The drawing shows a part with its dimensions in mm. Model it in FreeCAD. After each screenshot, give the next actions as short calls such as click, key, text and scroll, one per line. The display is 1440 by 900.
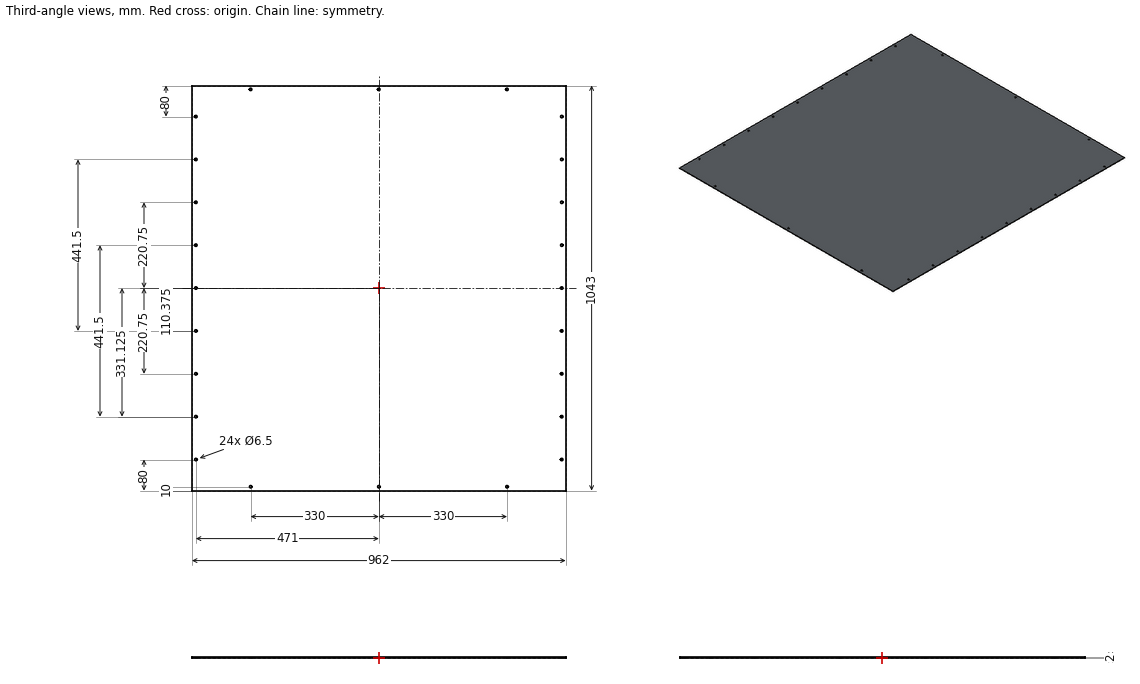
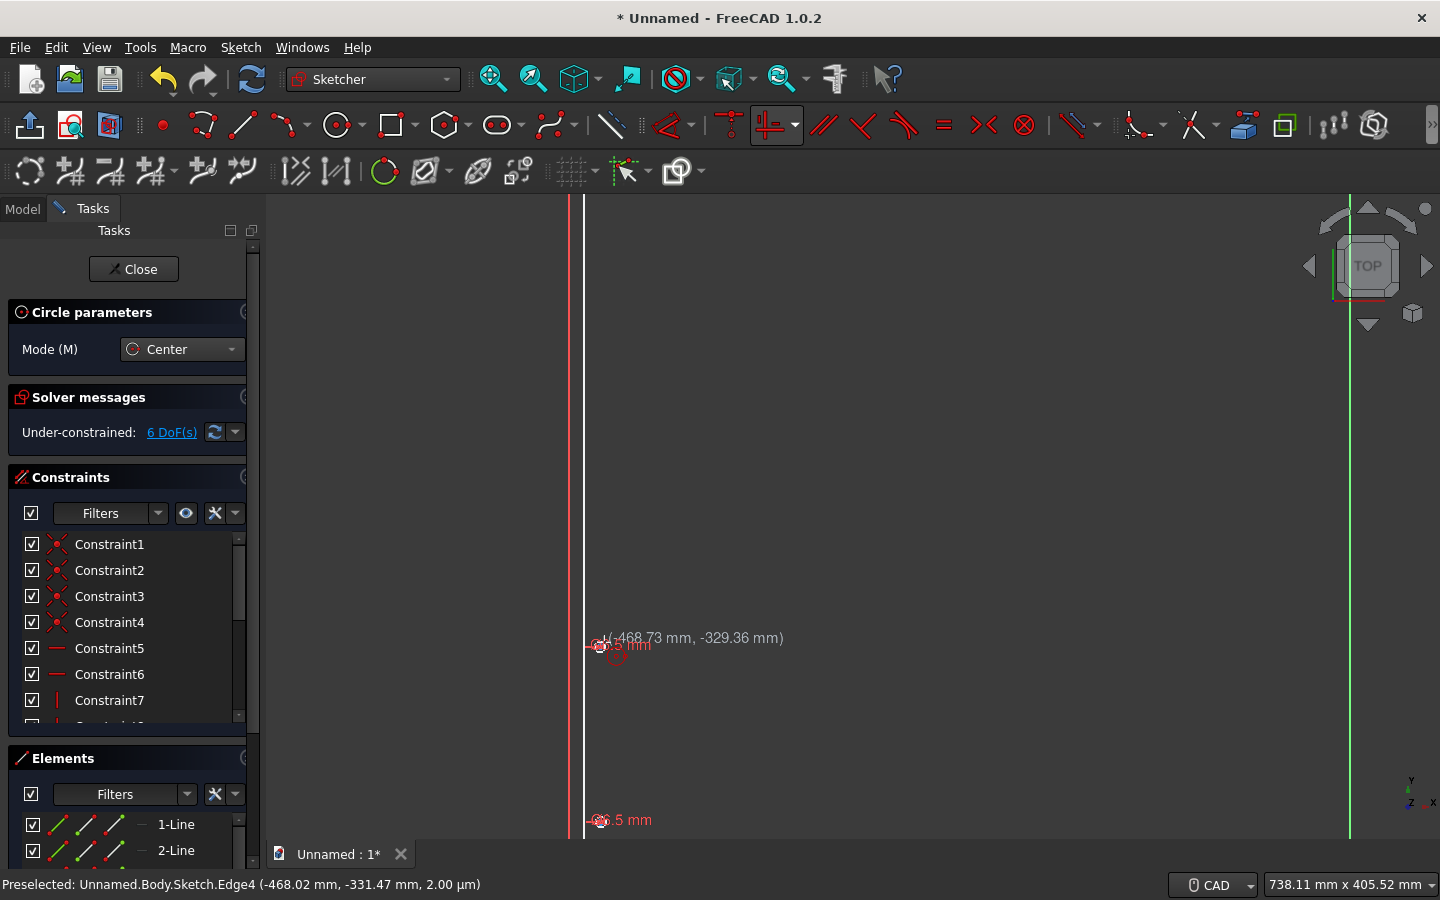
scroll(600, 470, up, 8)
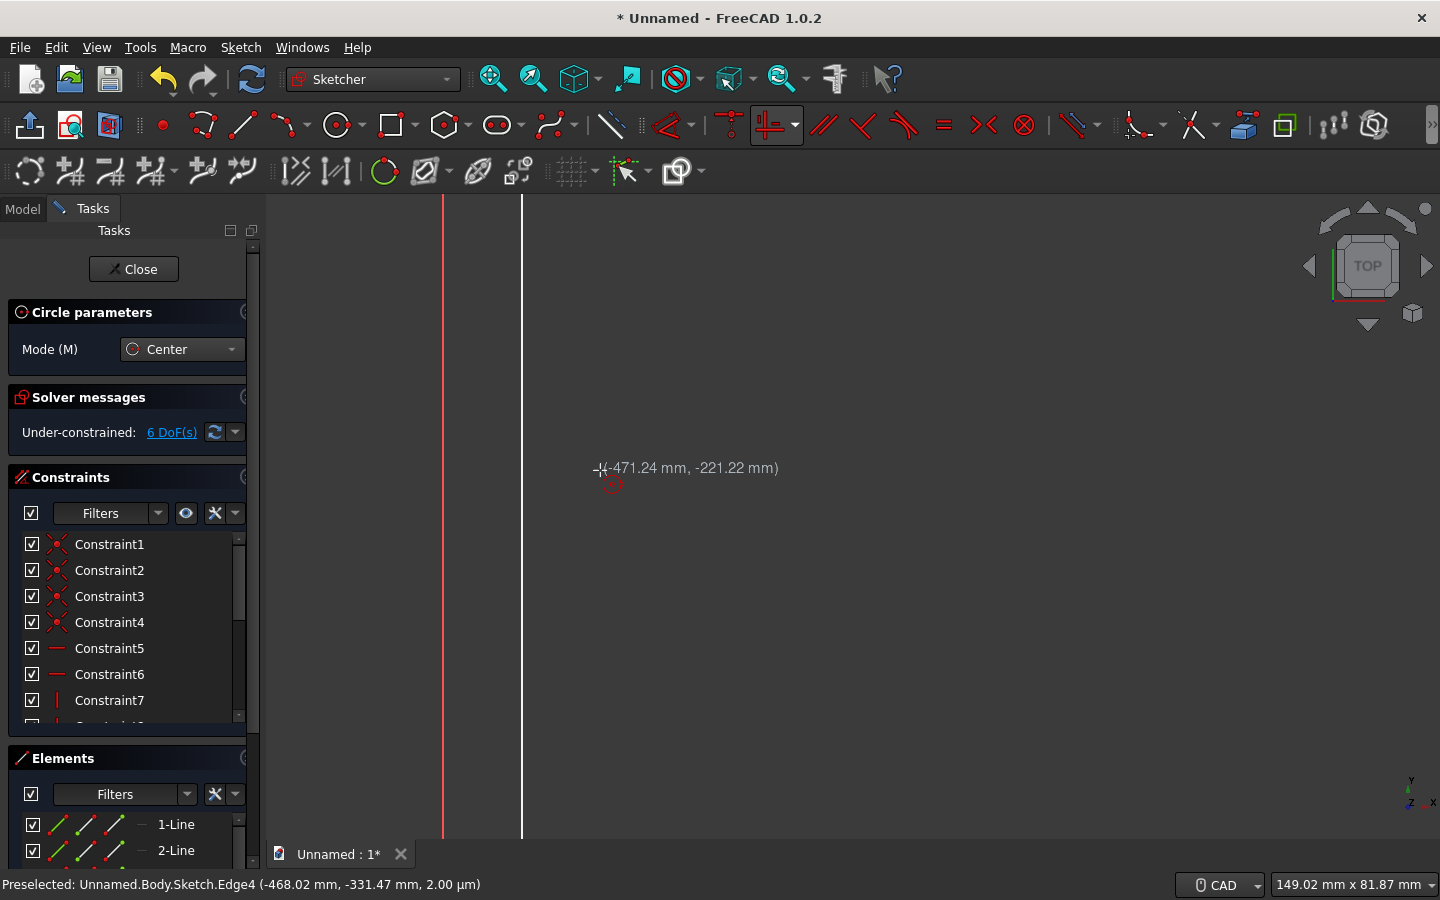
scroll(600, 610, down, 15)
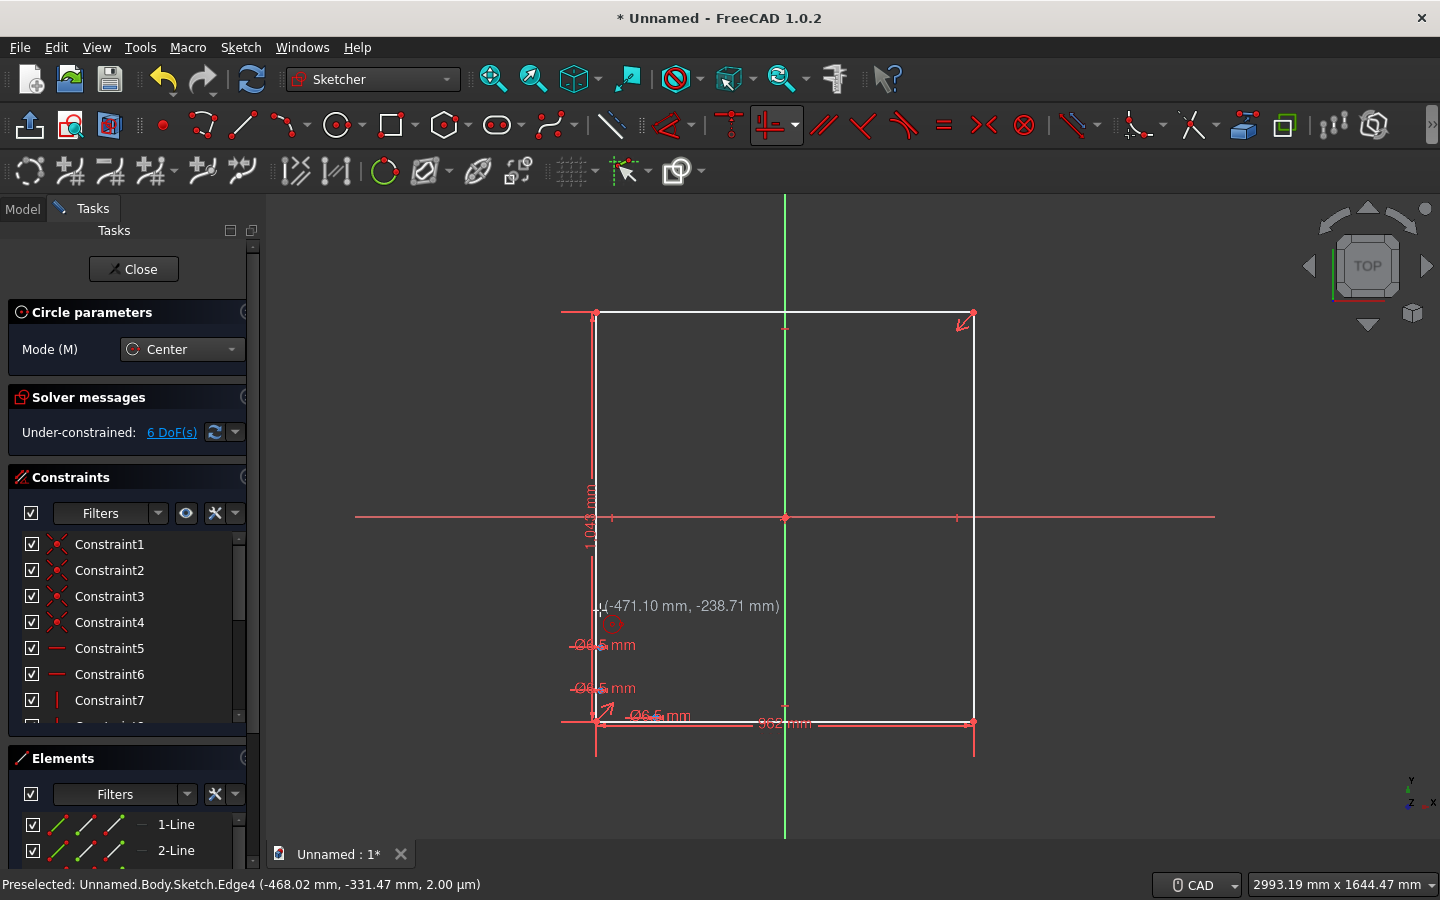
scroll(600, 604, up, 7)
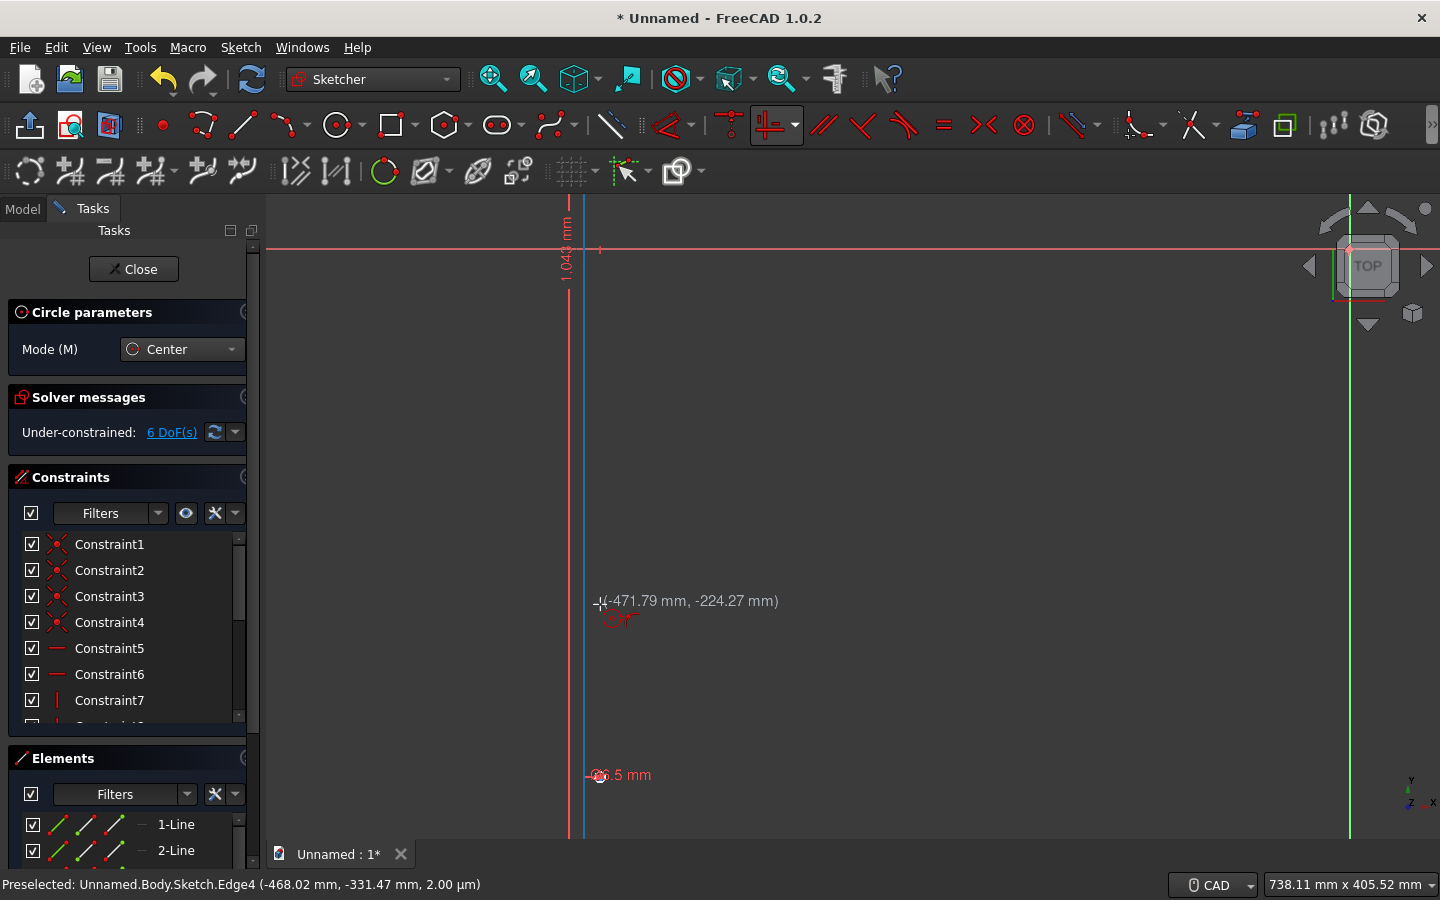
click(600, 601)
move(604, 597)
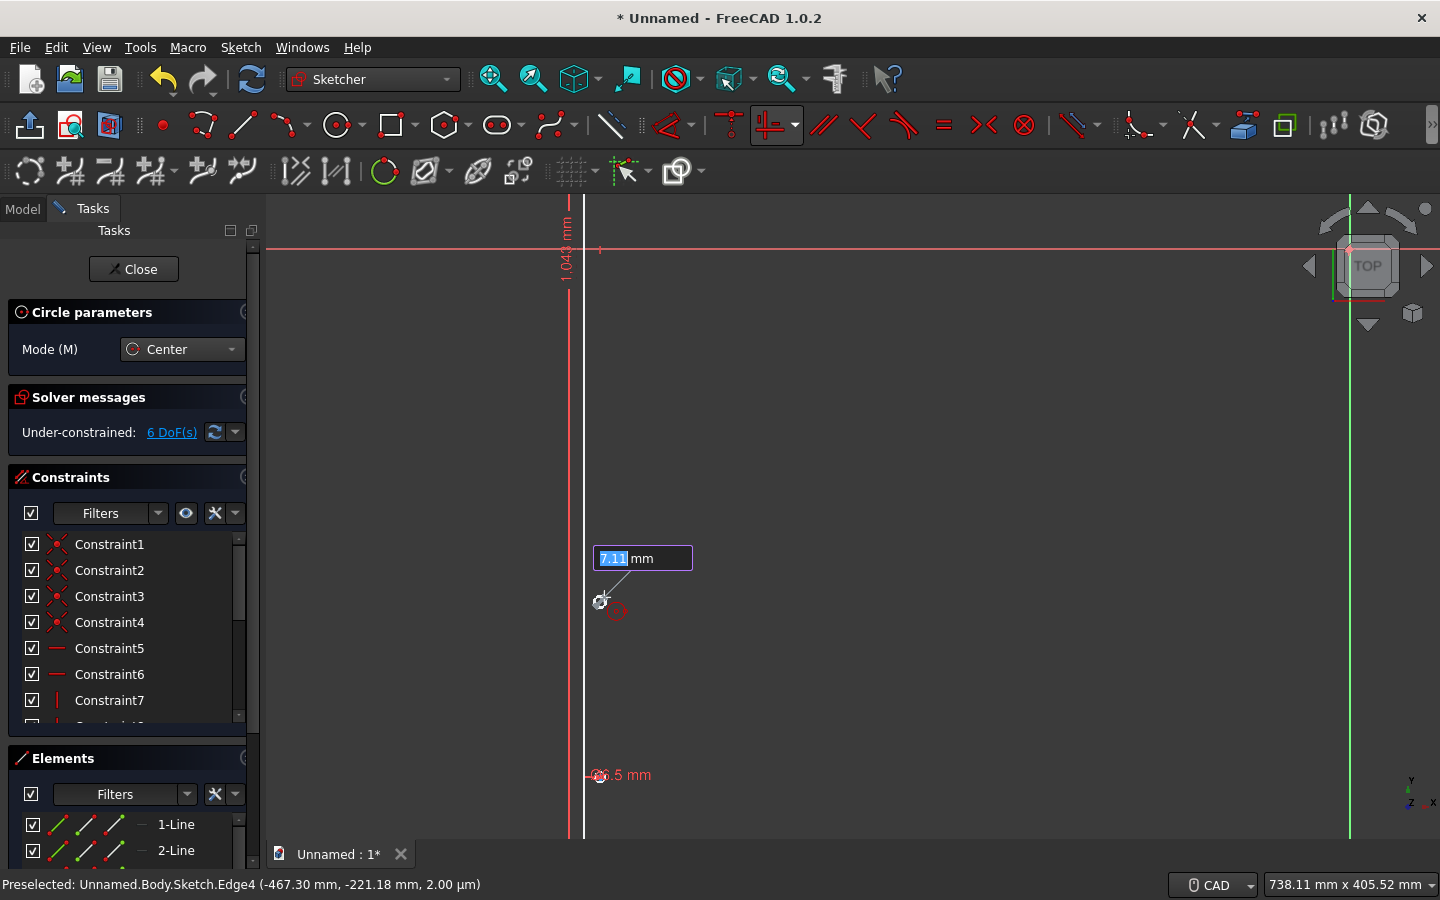
text(6.5)
key(Return)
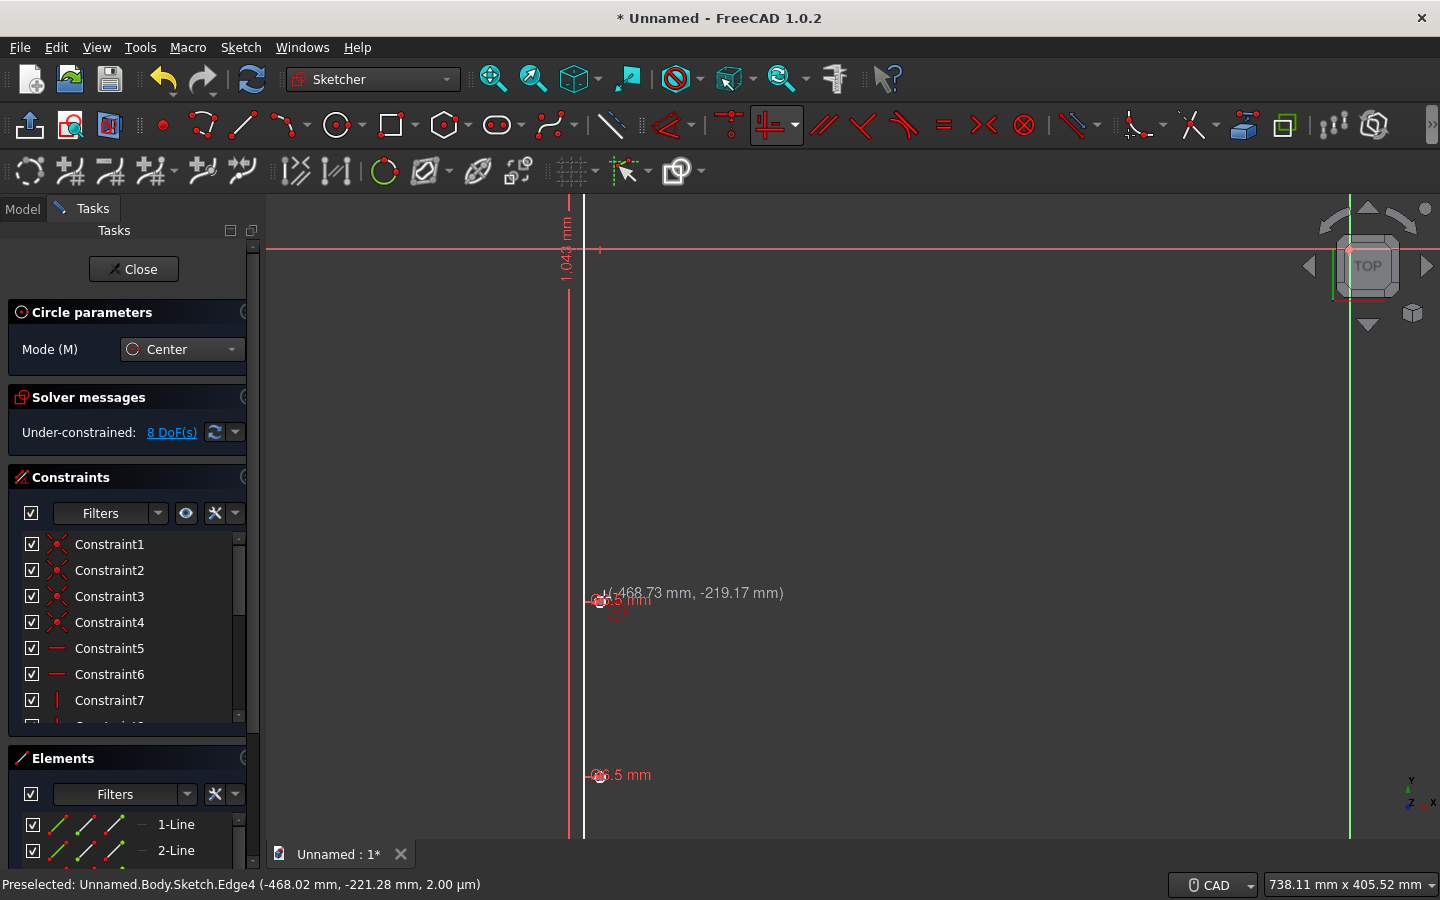
scroll(600, 425, up, 8)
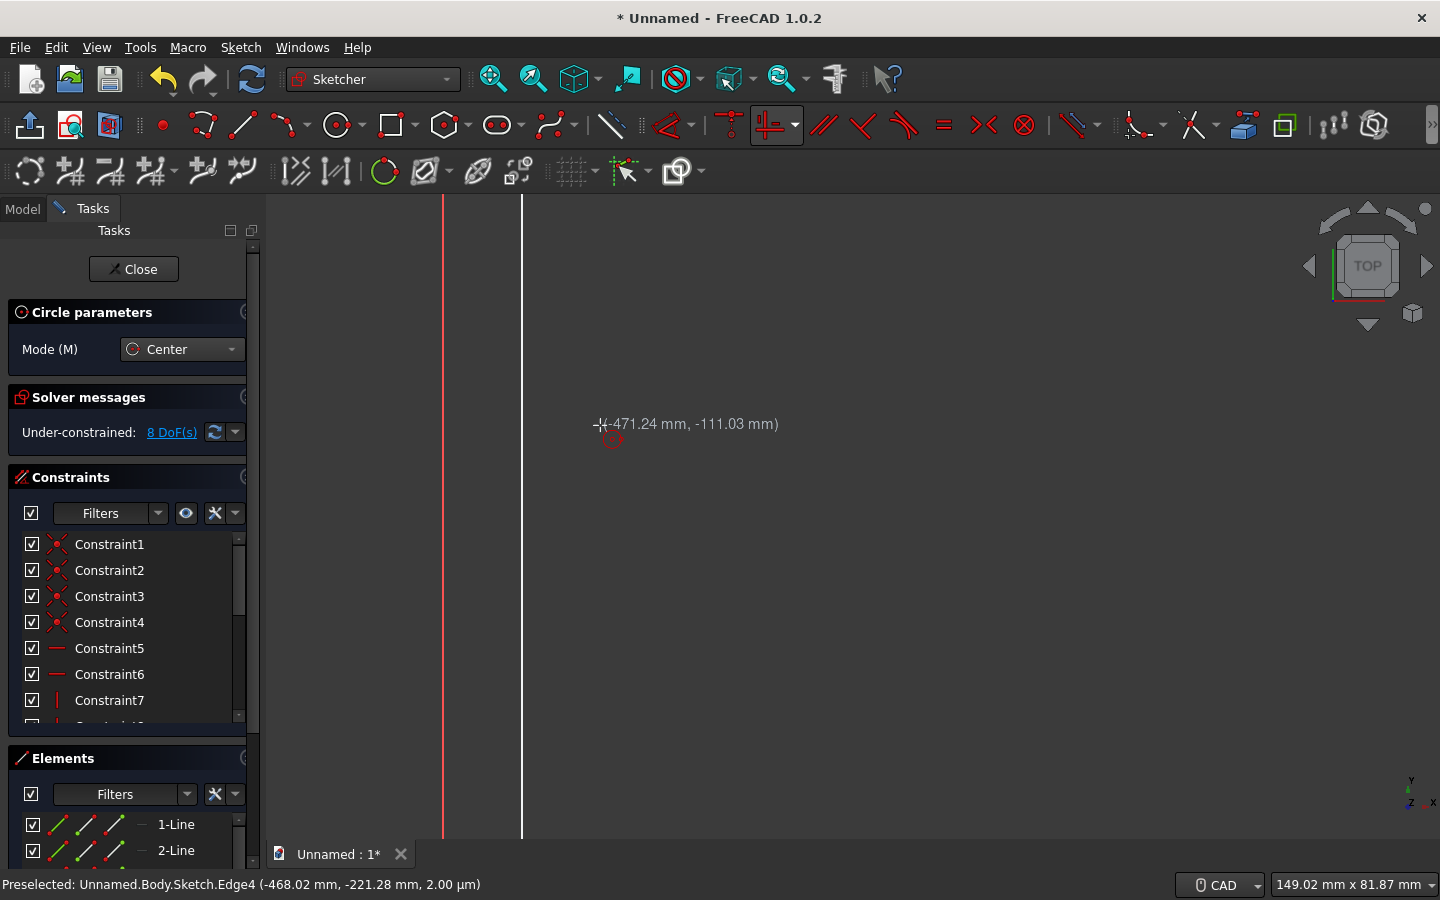
scroll(600, 567, down, 15)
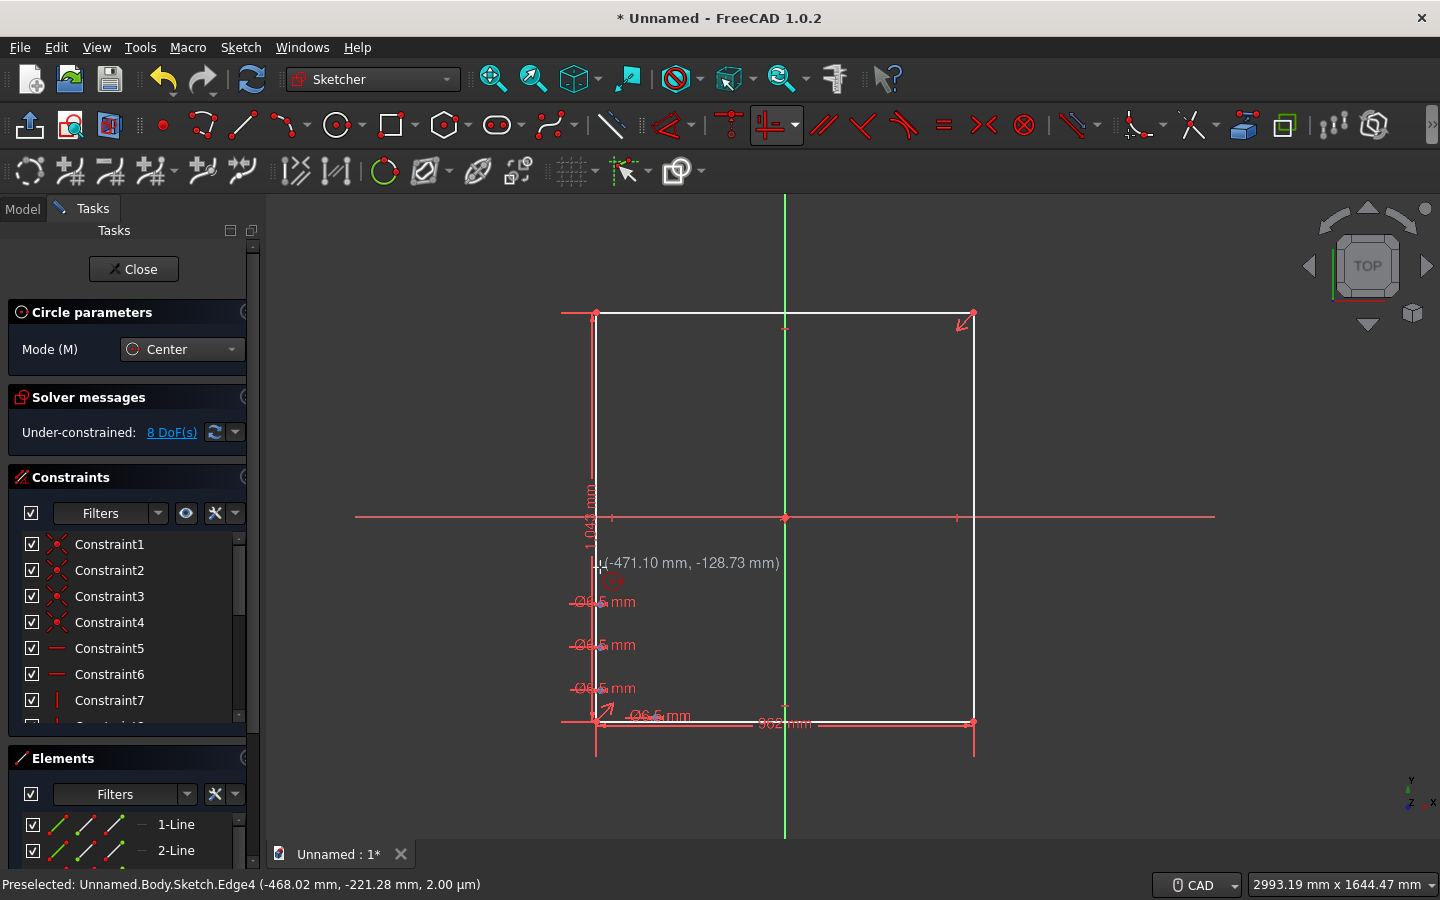
scroll(600, 560, up, 7)